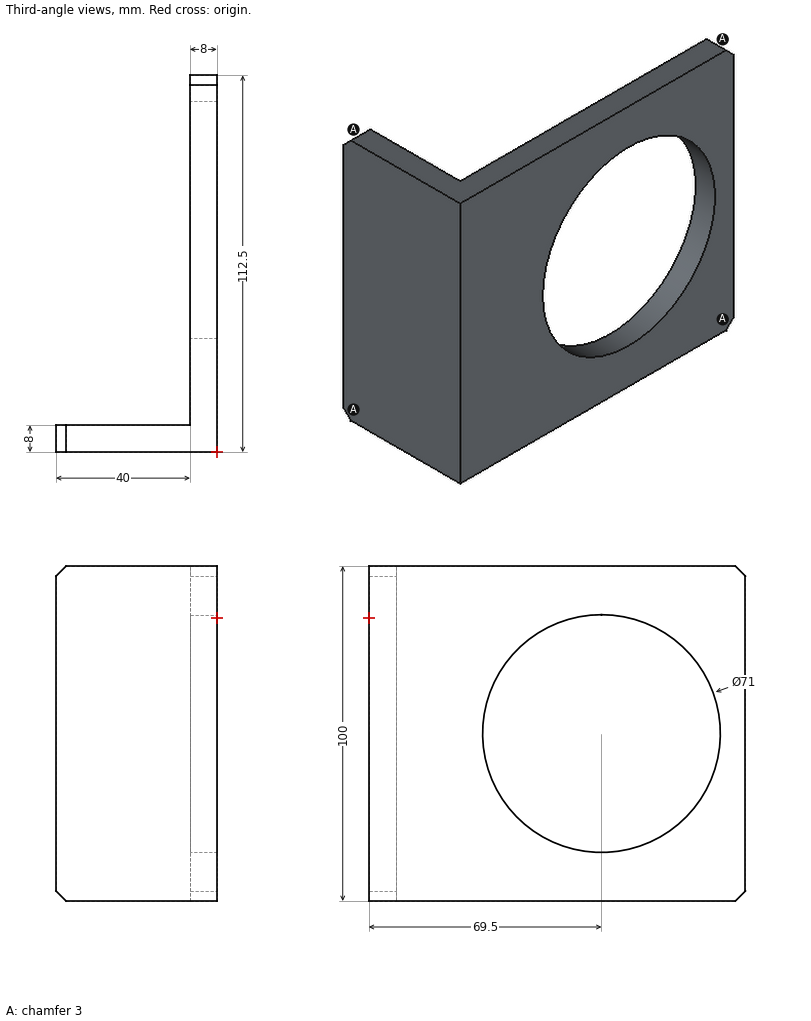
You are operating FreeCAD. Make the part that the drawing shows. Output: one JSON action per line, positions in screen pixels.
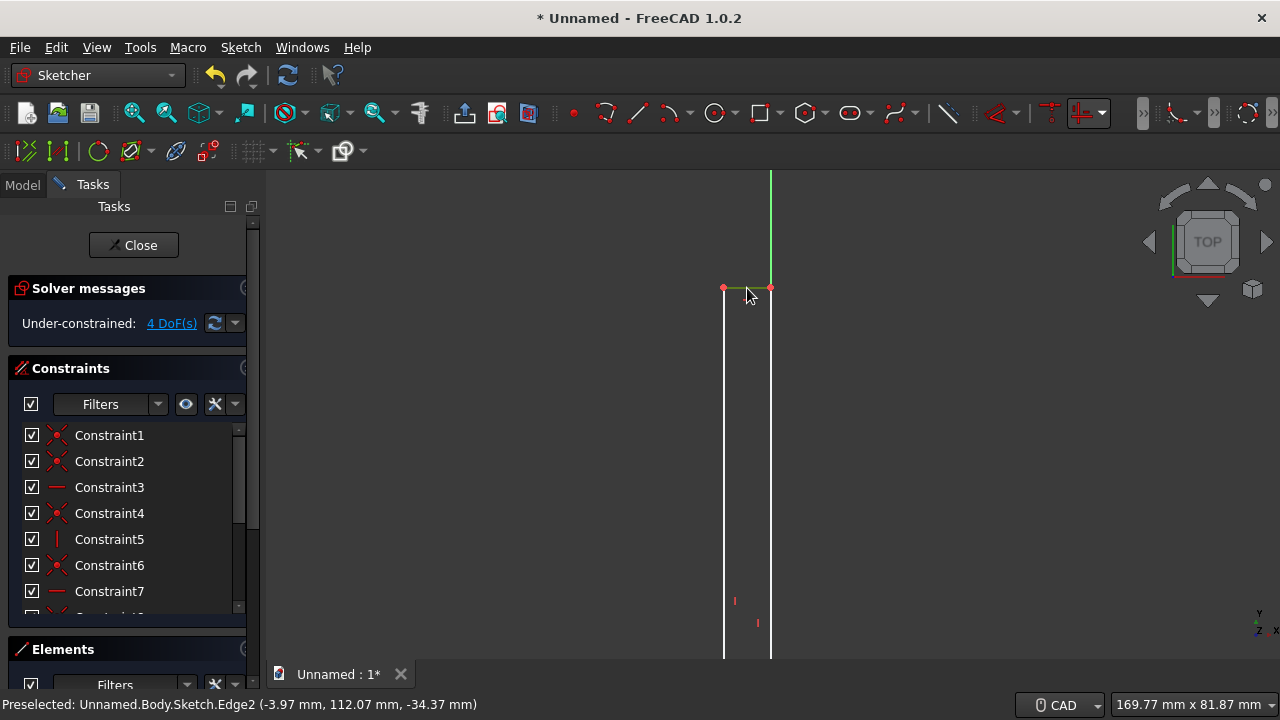
{"action": "left_click", "coordinate": [1018, 114]}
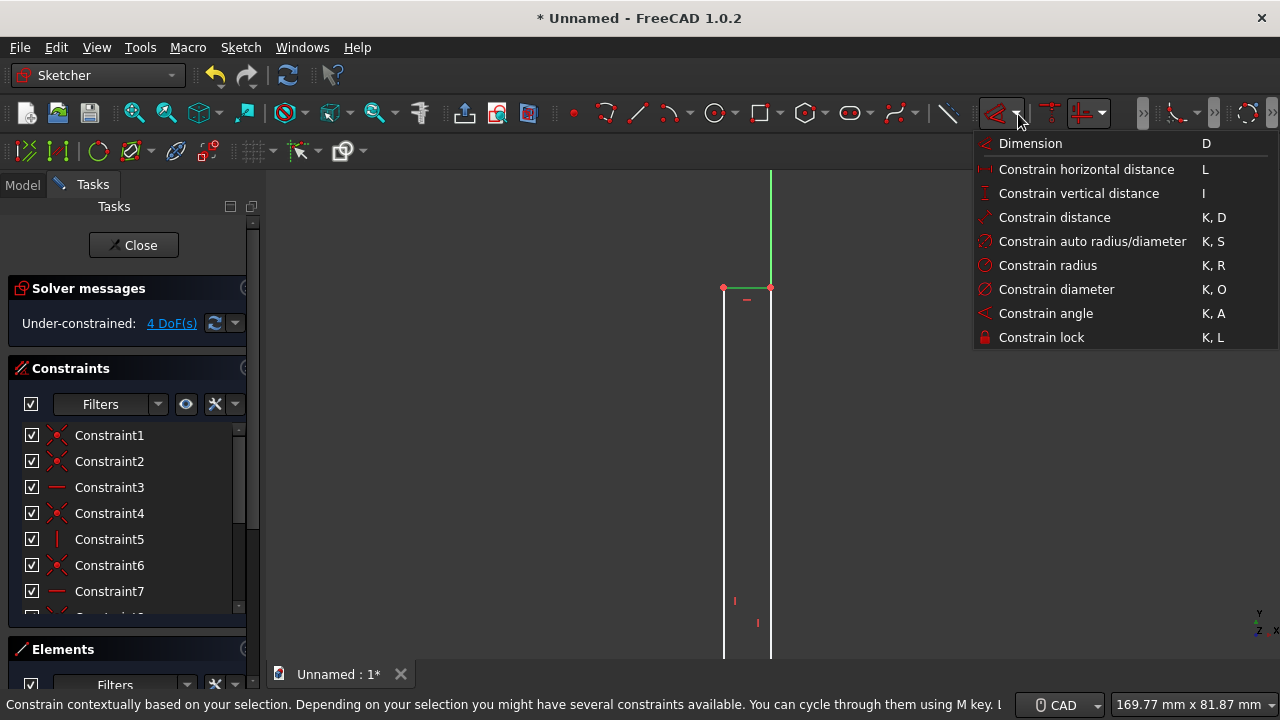
{"action": "left_click", "coordinate": [1126, 169]}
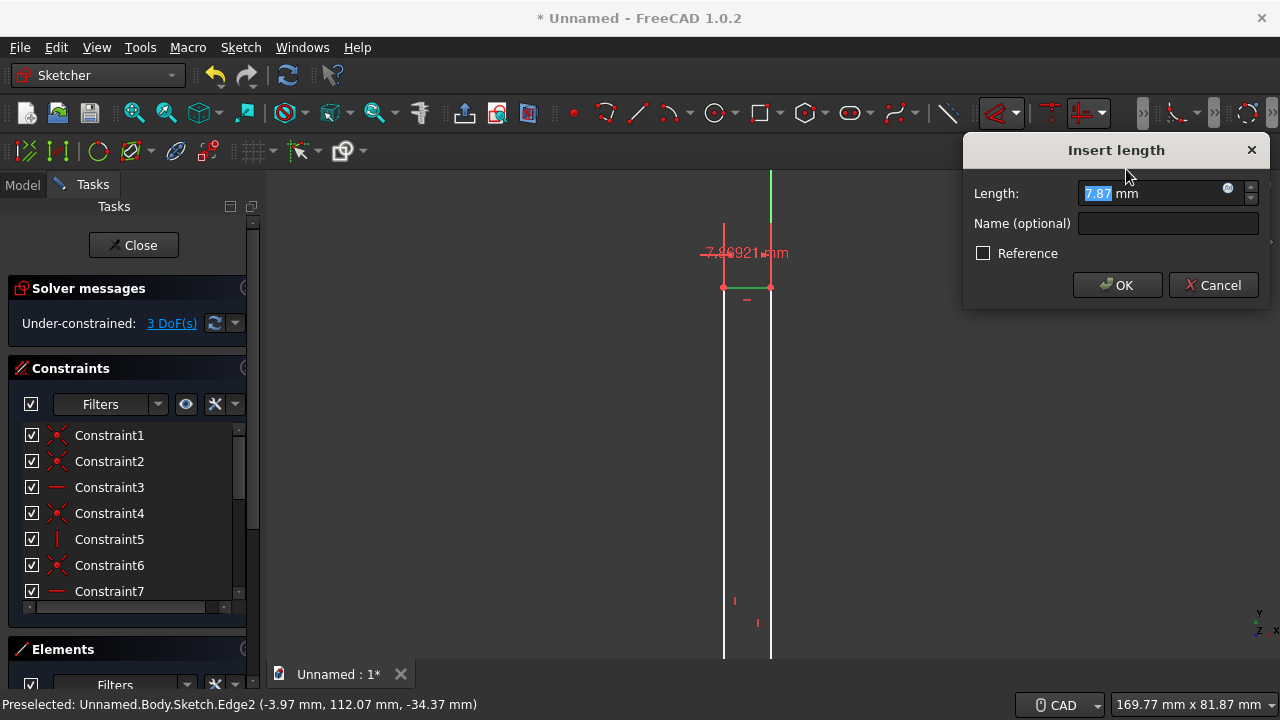
{"action": "type", "text": "8"}
{"action": "key", "text": "Return"}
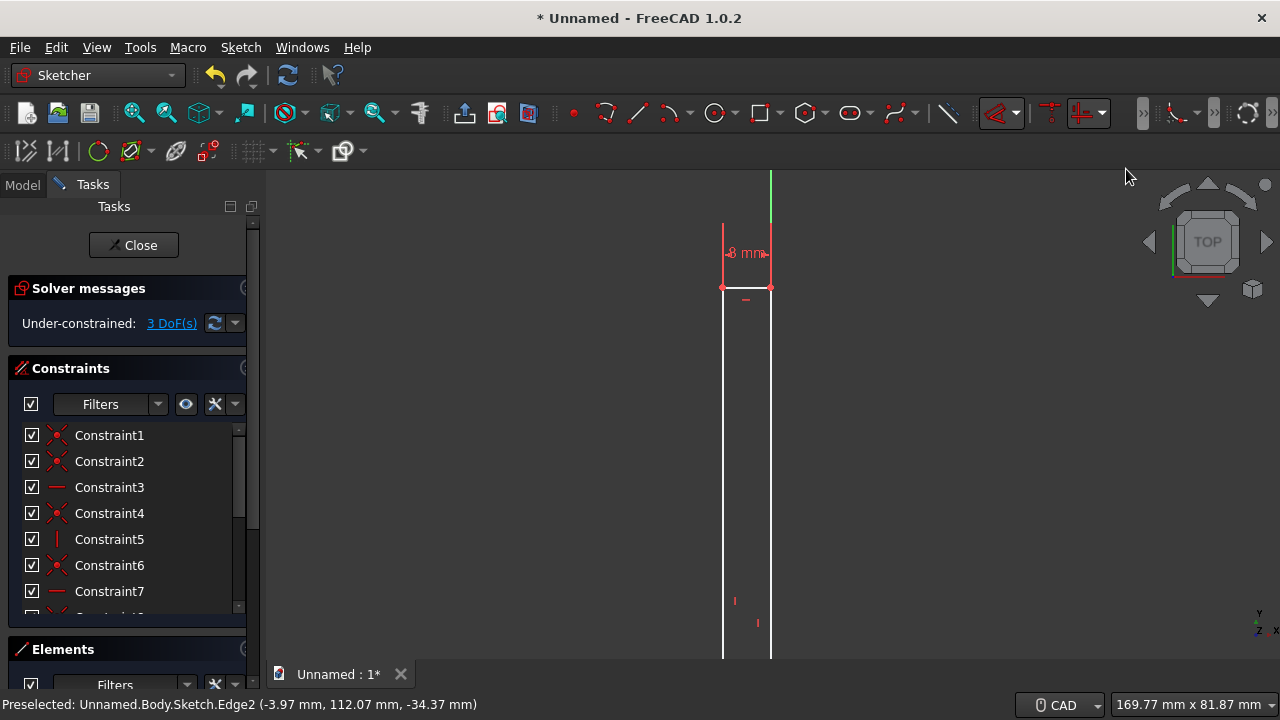
{"action": "scroll", "coordinate": [767, 246], "scroll_direction": "down", "scroll_amount": 4}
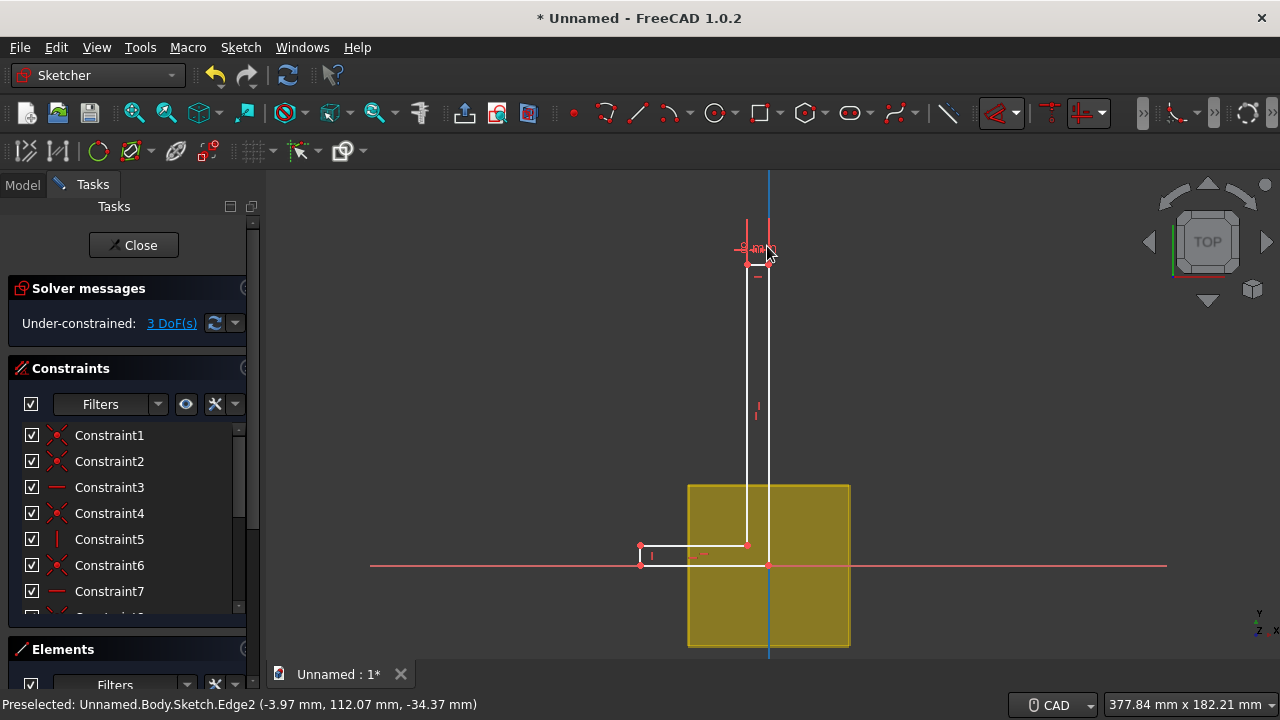
{"action": "scroll", "coordinate": [640, 552], "scroll_direction": "up", "scroll_amount": 5}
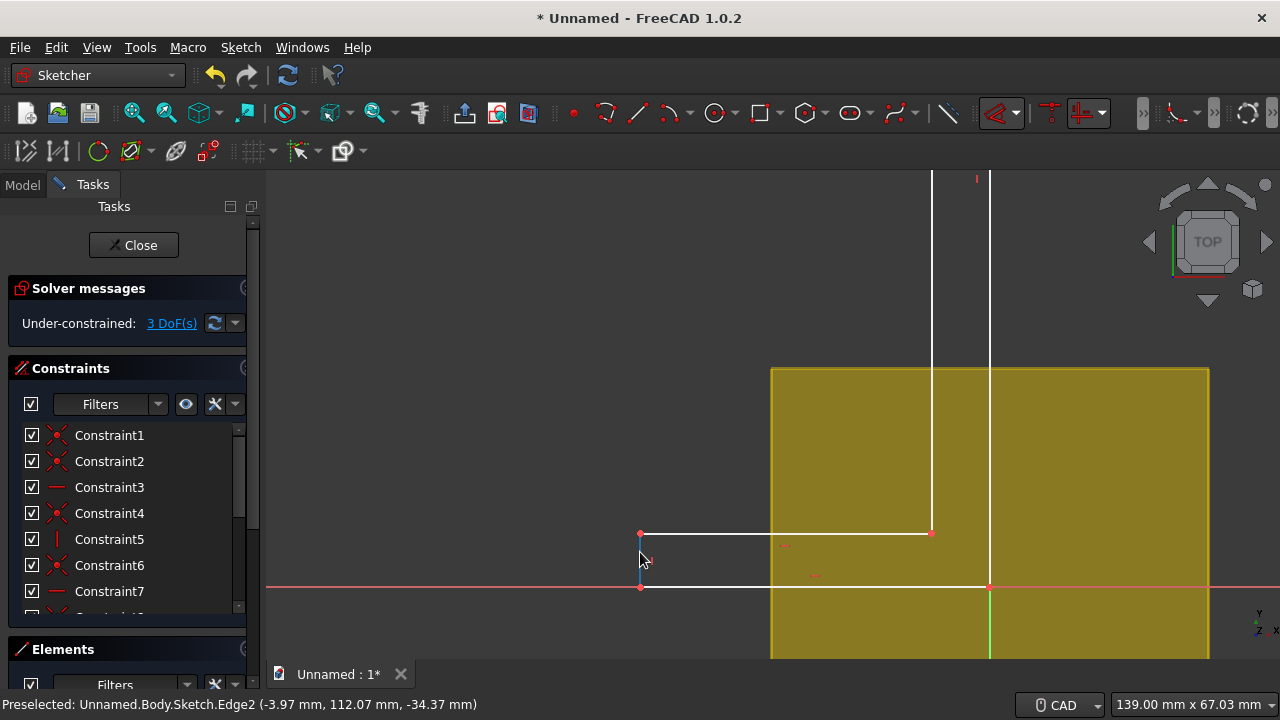
{"action": "left_click", "coordinate": [640, 550]}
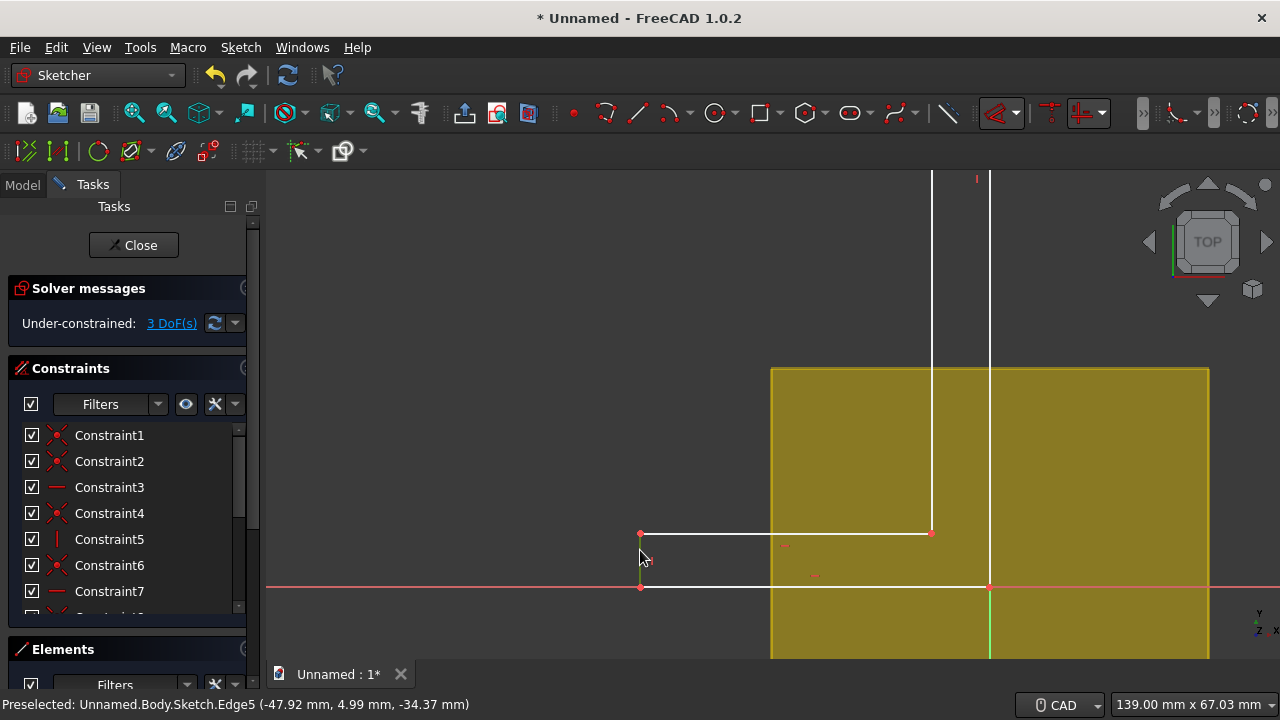
{"action": "left_click", "coordinate": [1018, 114]}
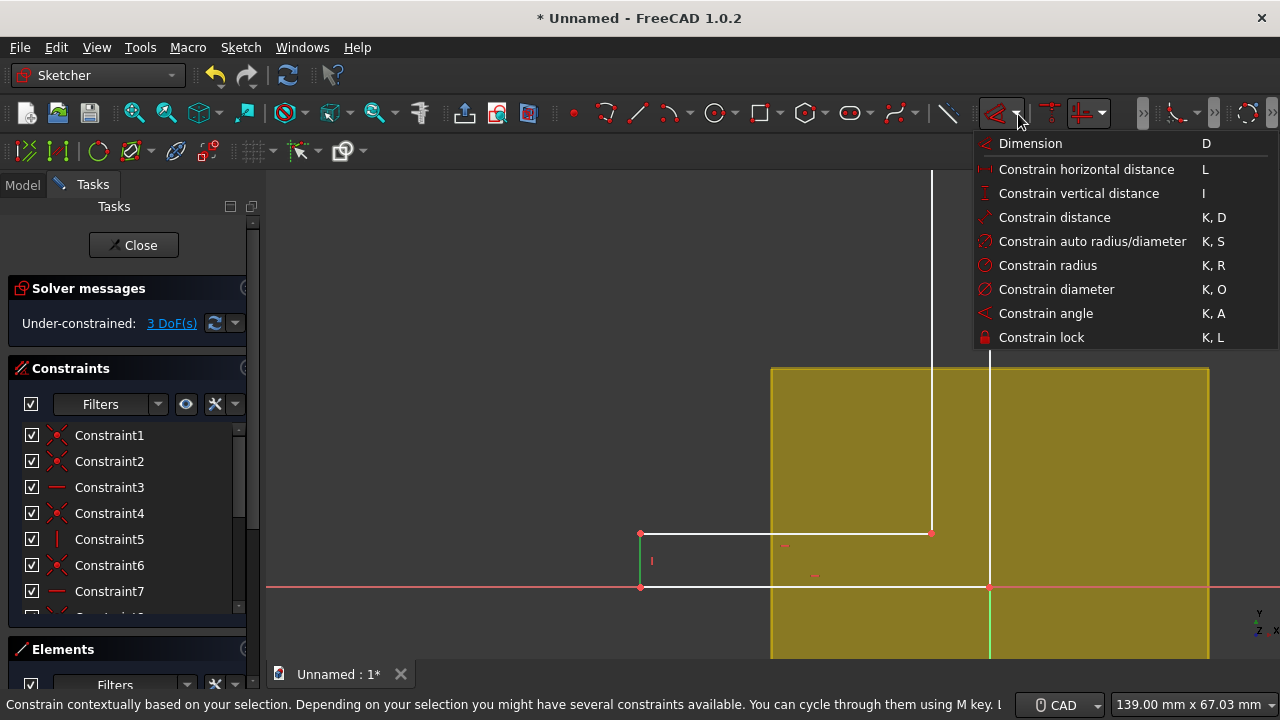
{"action": "left_click", "coordinate": [1126, 193]}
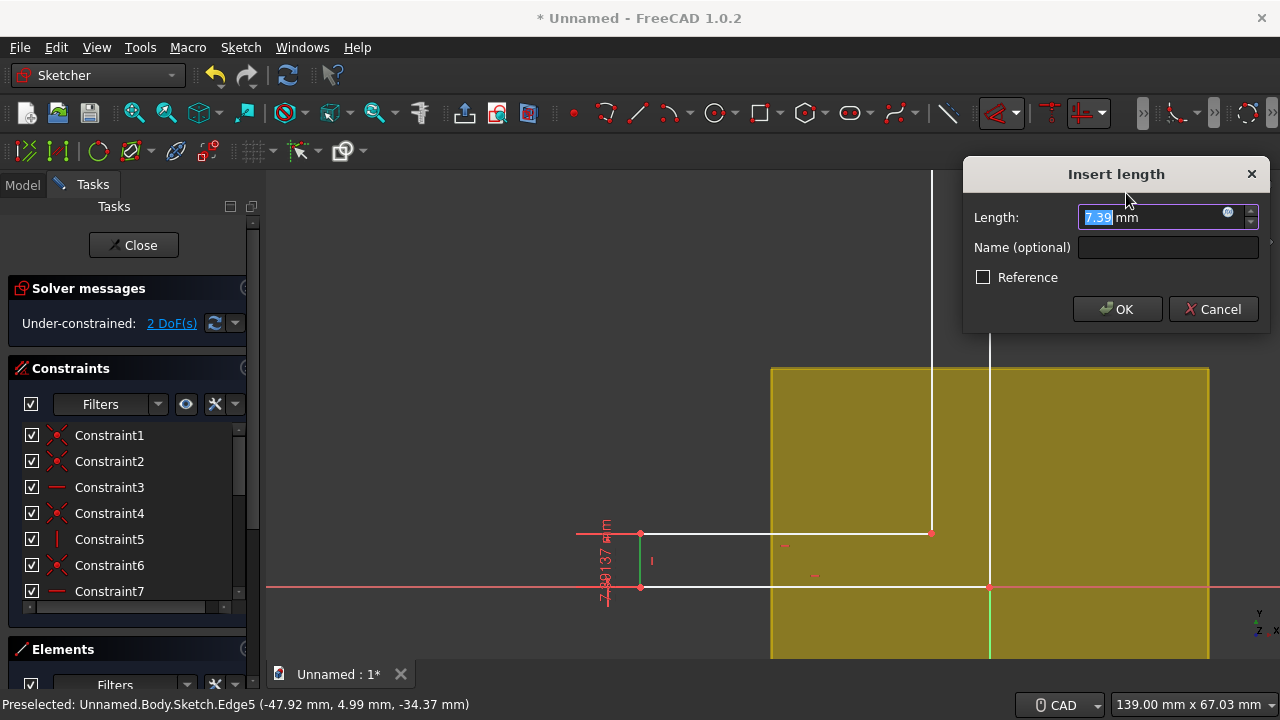
{"action": "type", "text": "8"}
{"action": "key", "text": "Return"}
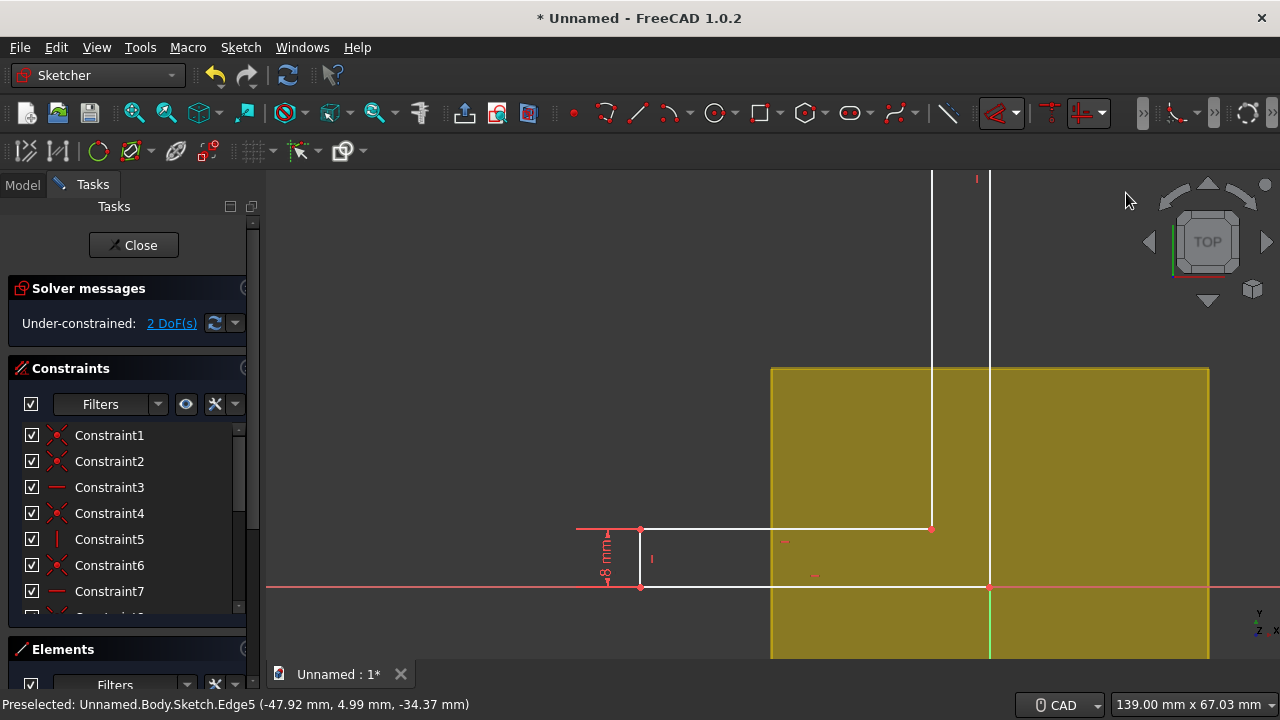
{"action": "left_click", "coordinate": [844, 529]}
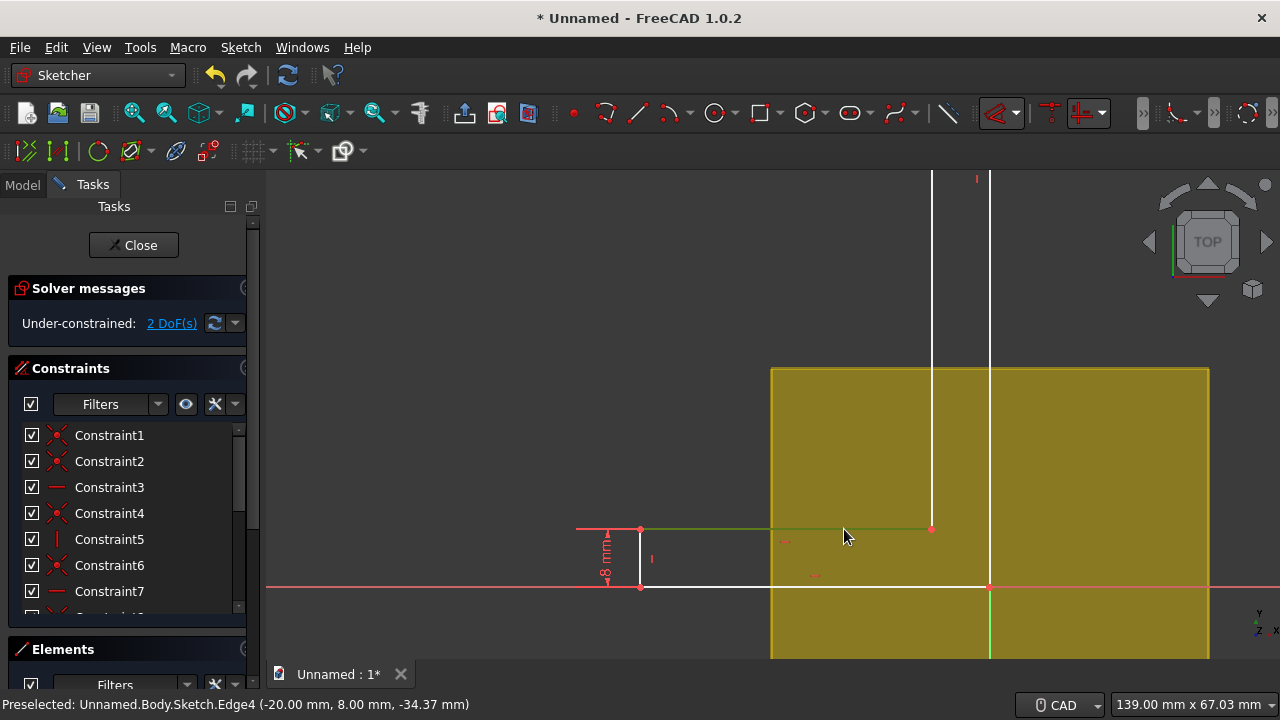
{"action": "left_click", "coordinate": [1018, 114]}